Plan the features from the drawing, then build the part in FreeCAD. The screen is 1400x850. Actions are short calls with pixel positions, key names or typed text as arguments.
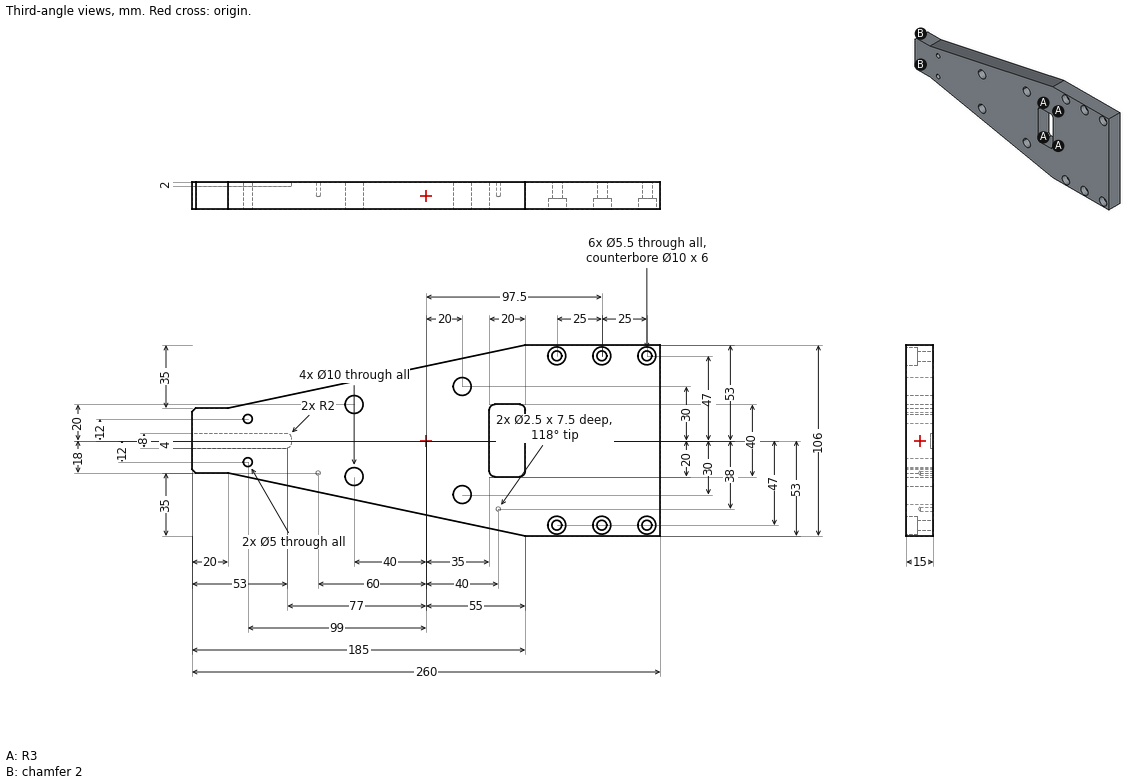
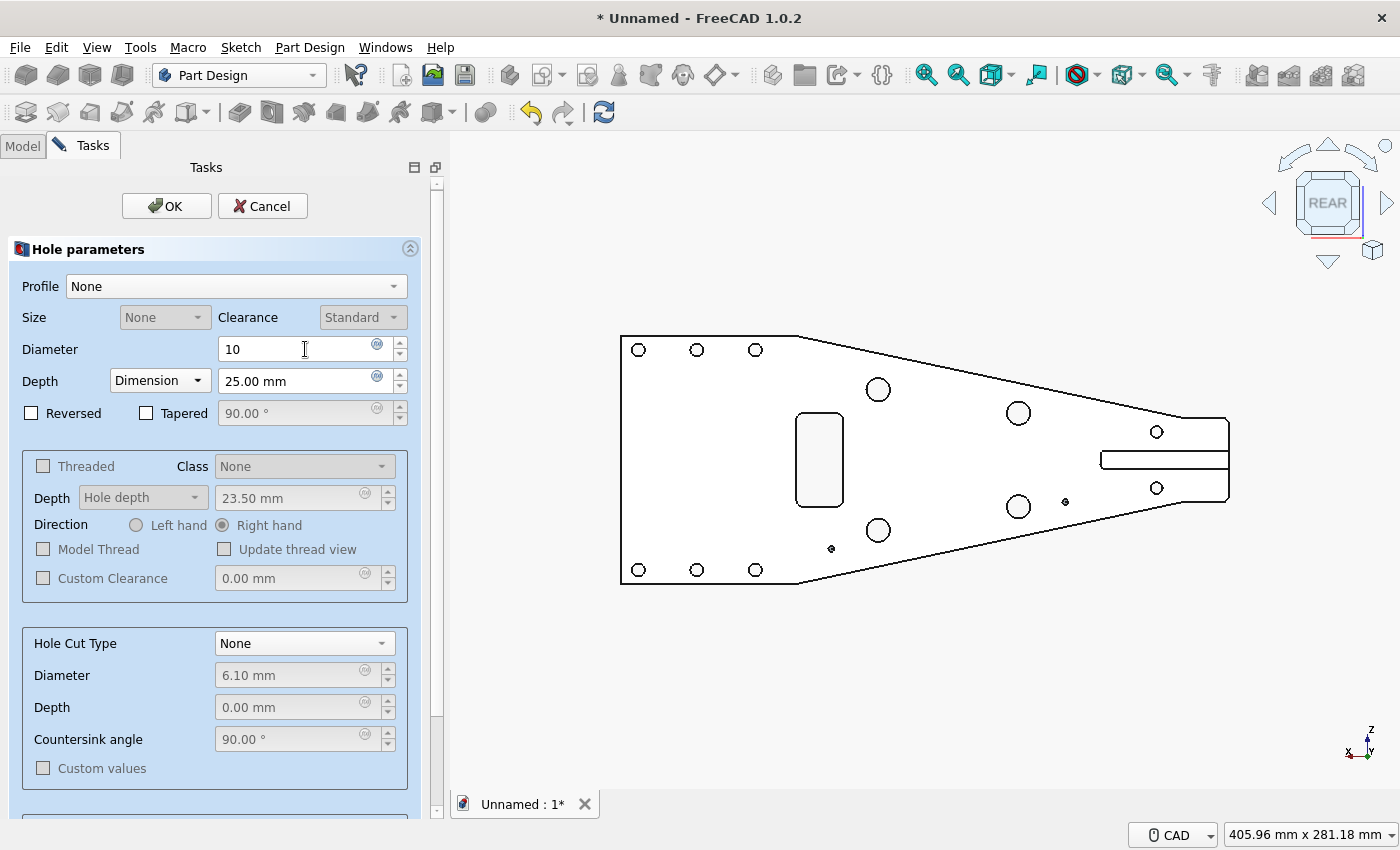
click(161, 380)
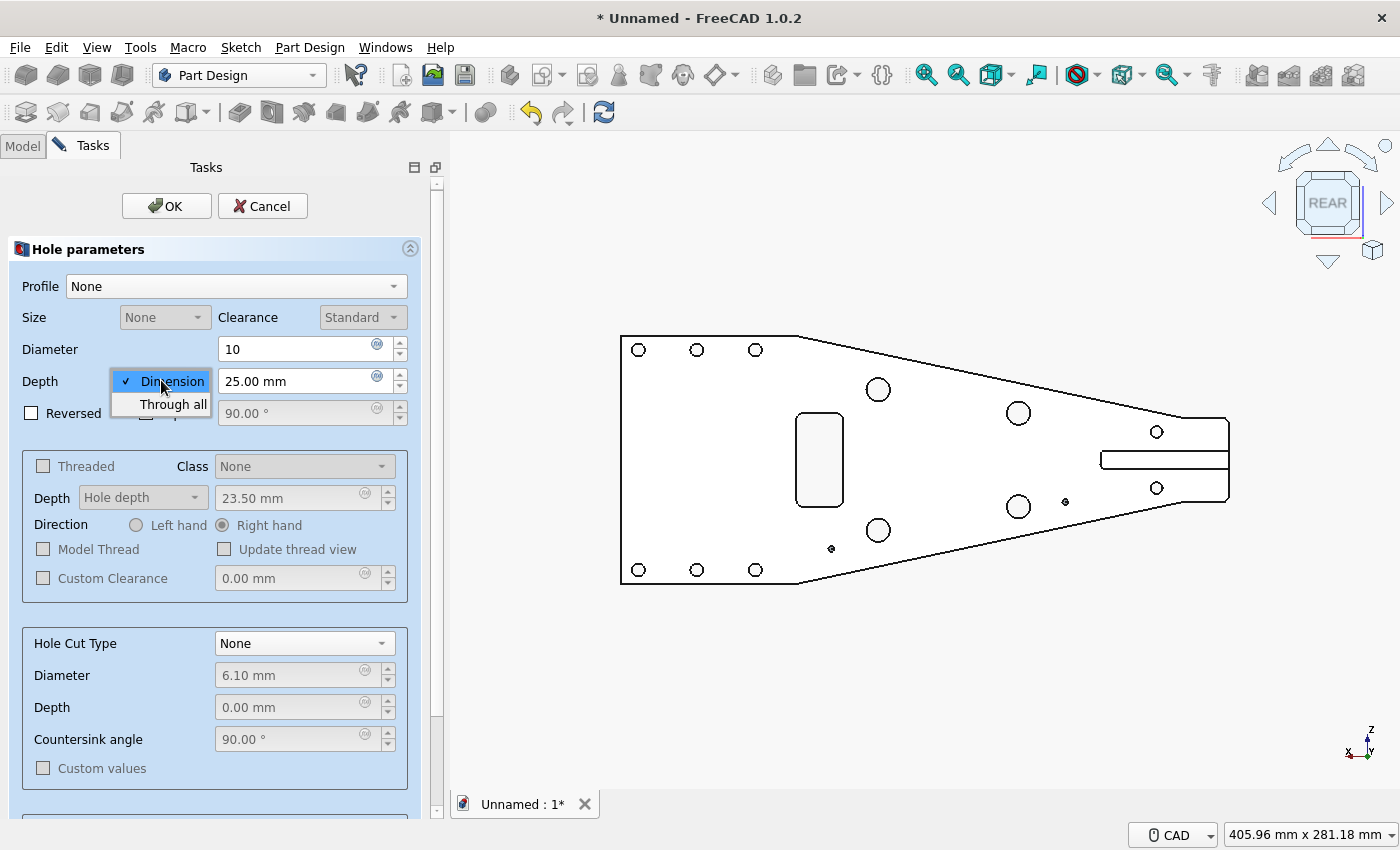
click(160, 404)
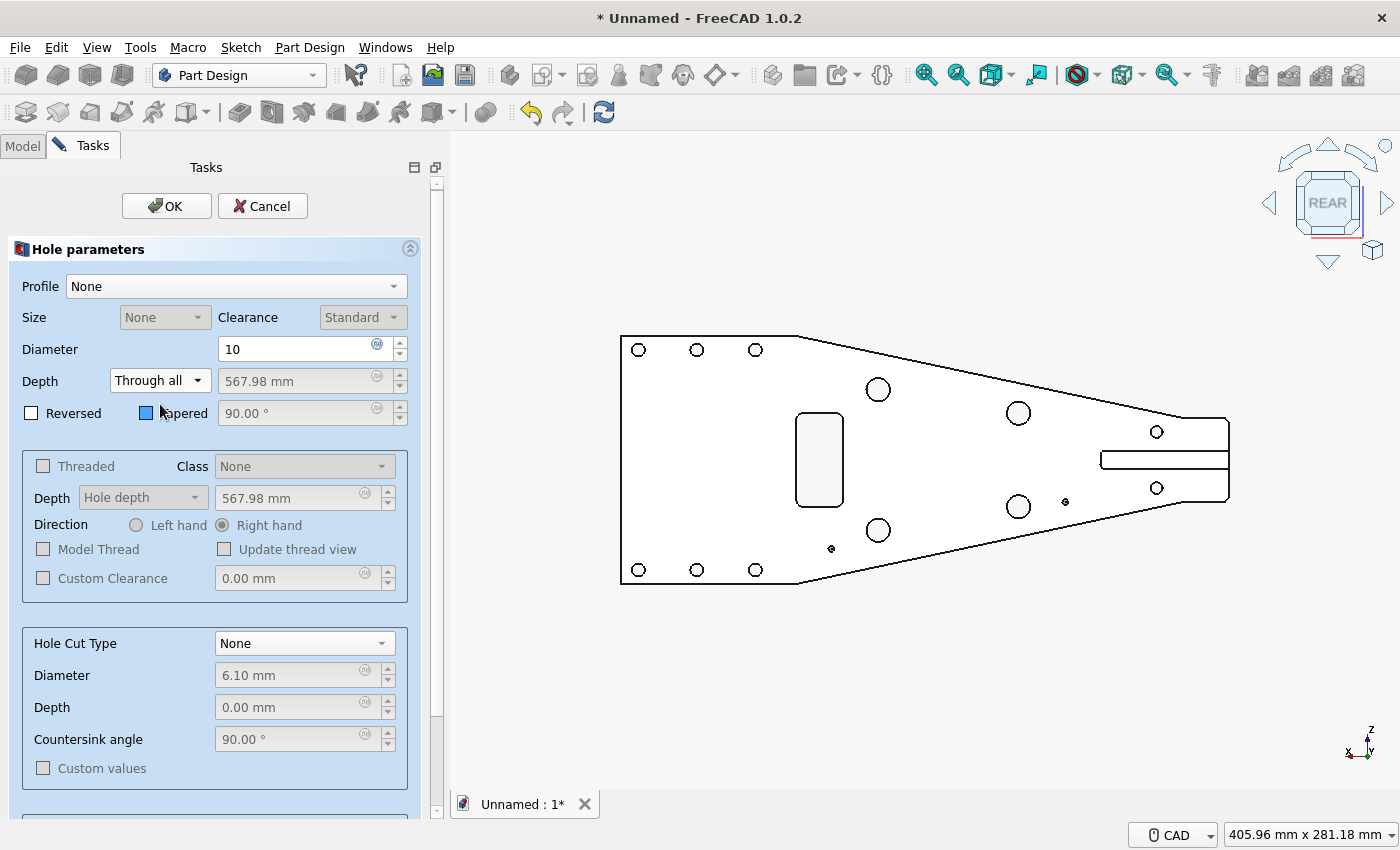
click(167, 206)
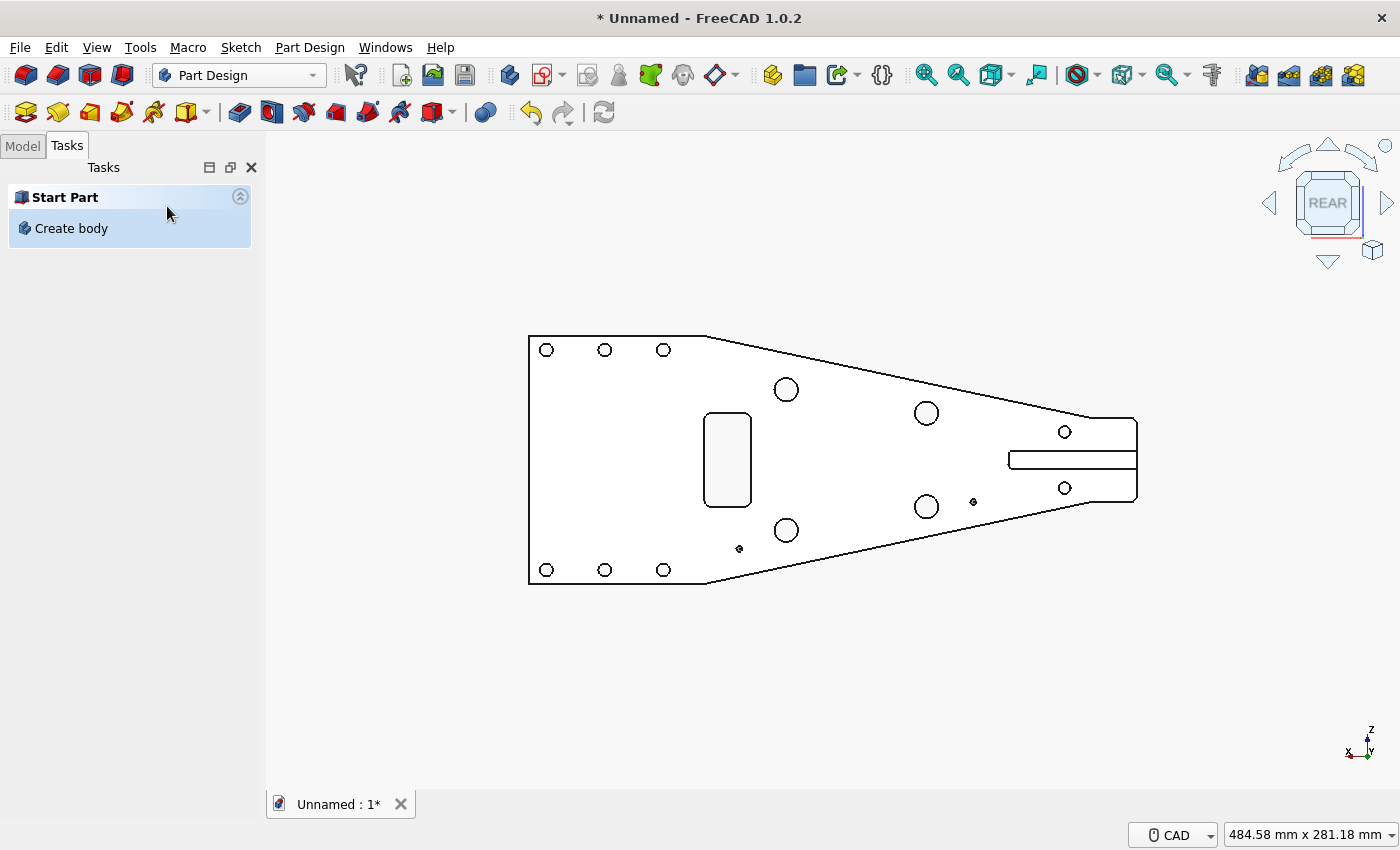
key(0)